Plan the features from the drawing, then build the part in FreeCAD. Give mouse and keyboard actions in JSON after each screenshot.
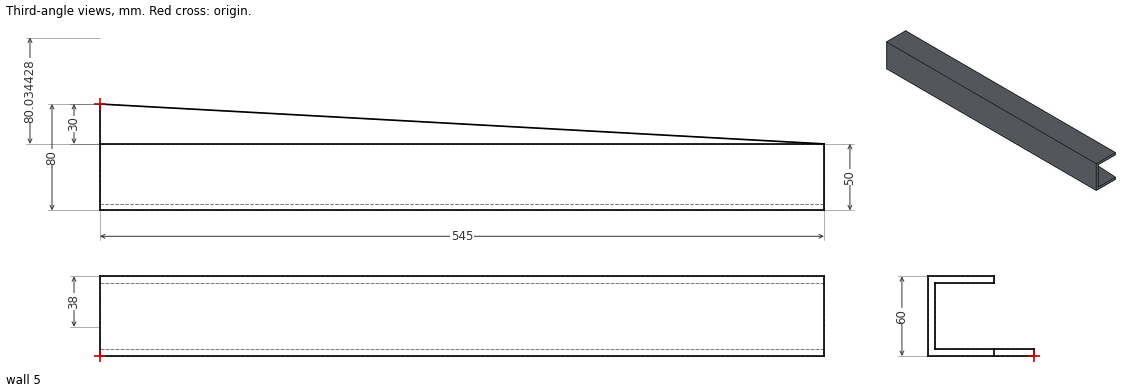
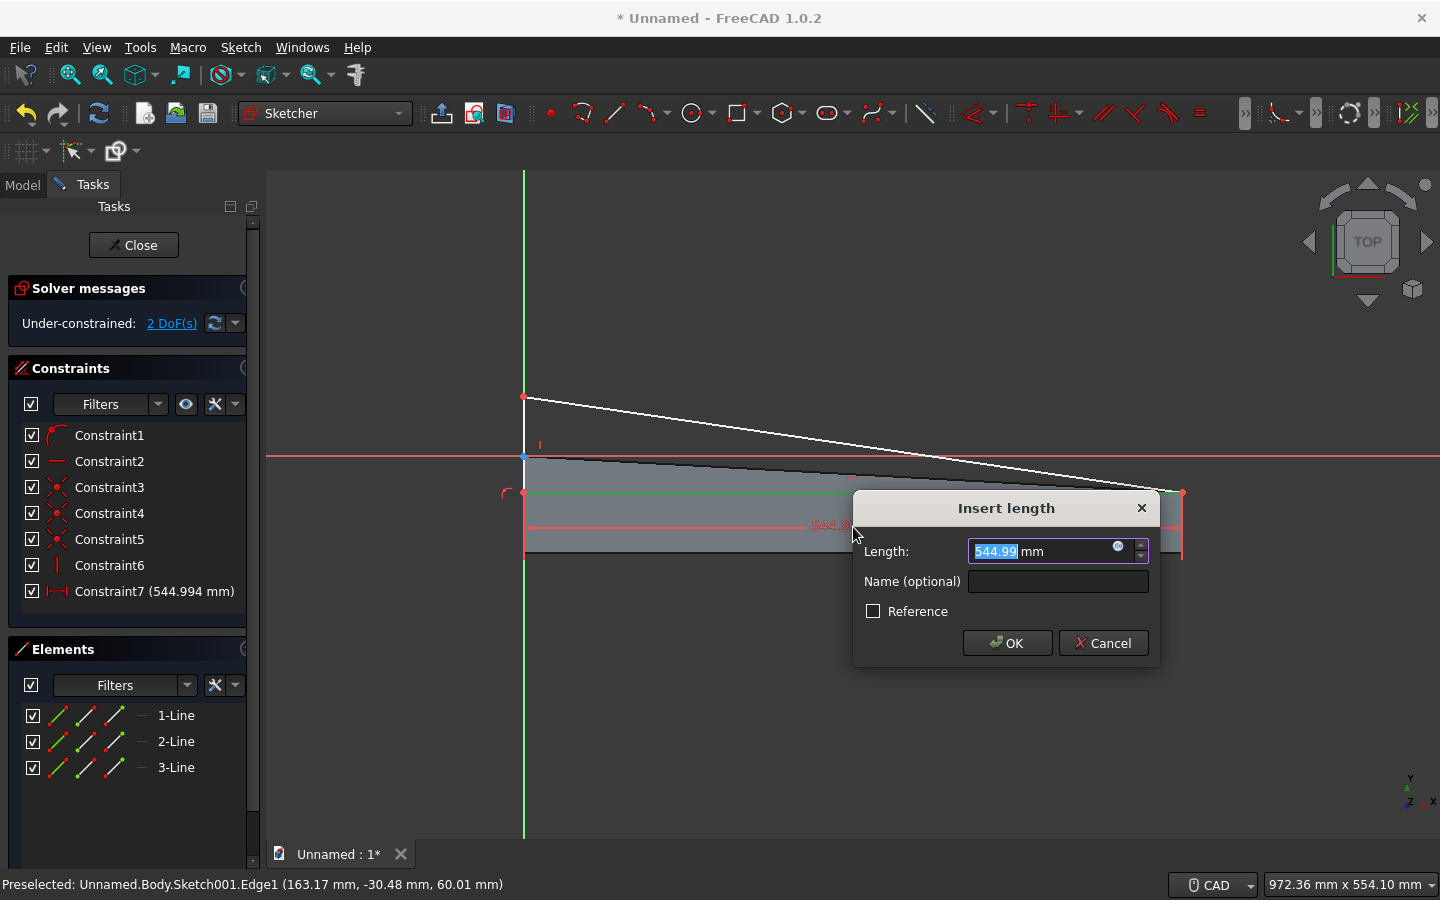
{"action": "type", "text": "545"}
{"action": "key", "text": "Return"}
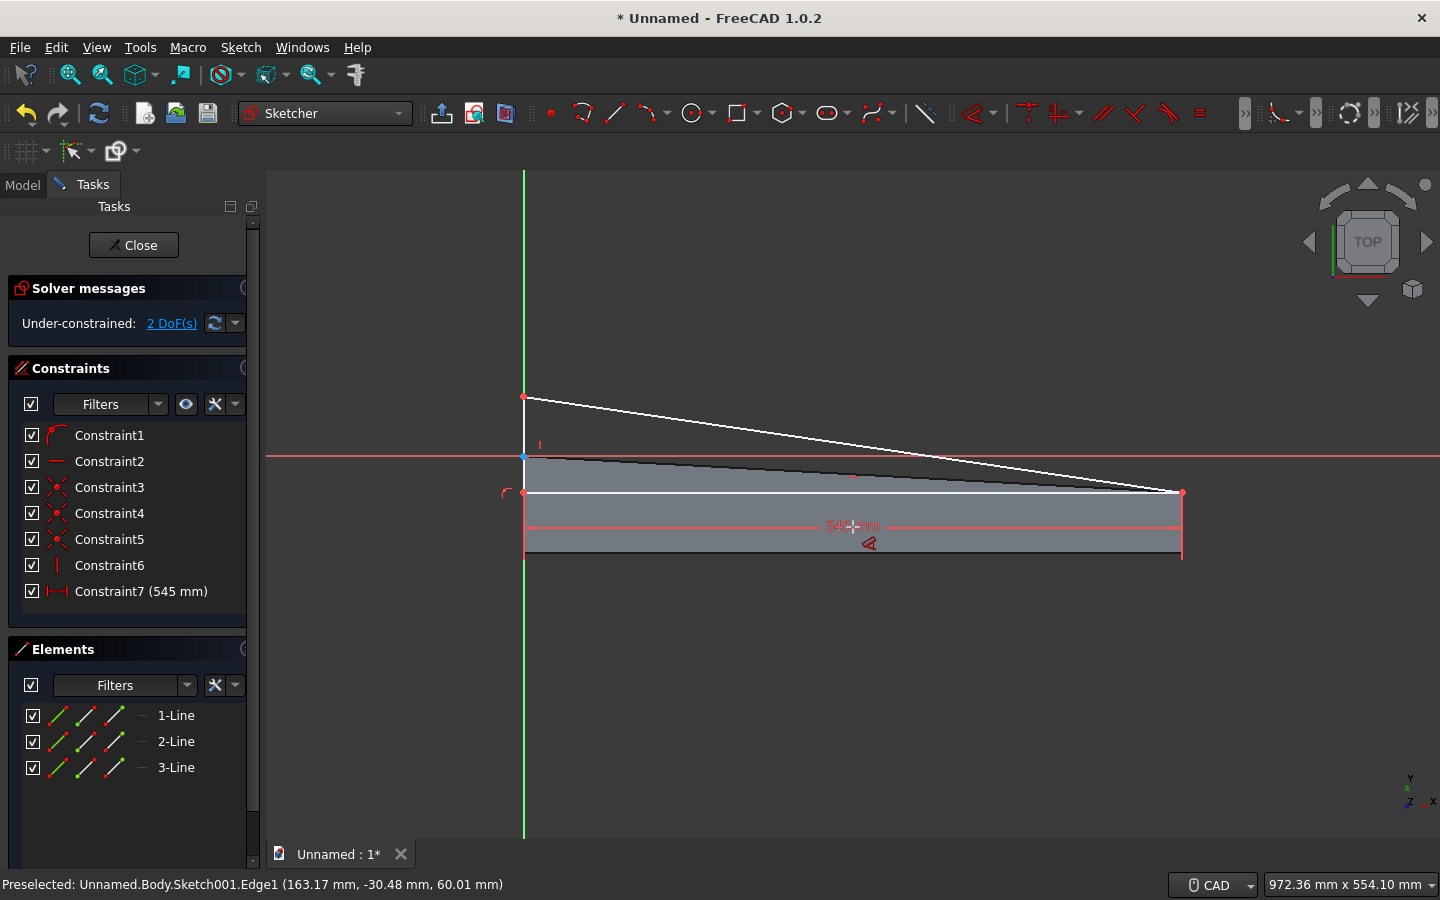
{"action": "left_click", "coordinate": [524, 493]}
{"action": "left_click", "coordinate": [490, 475]}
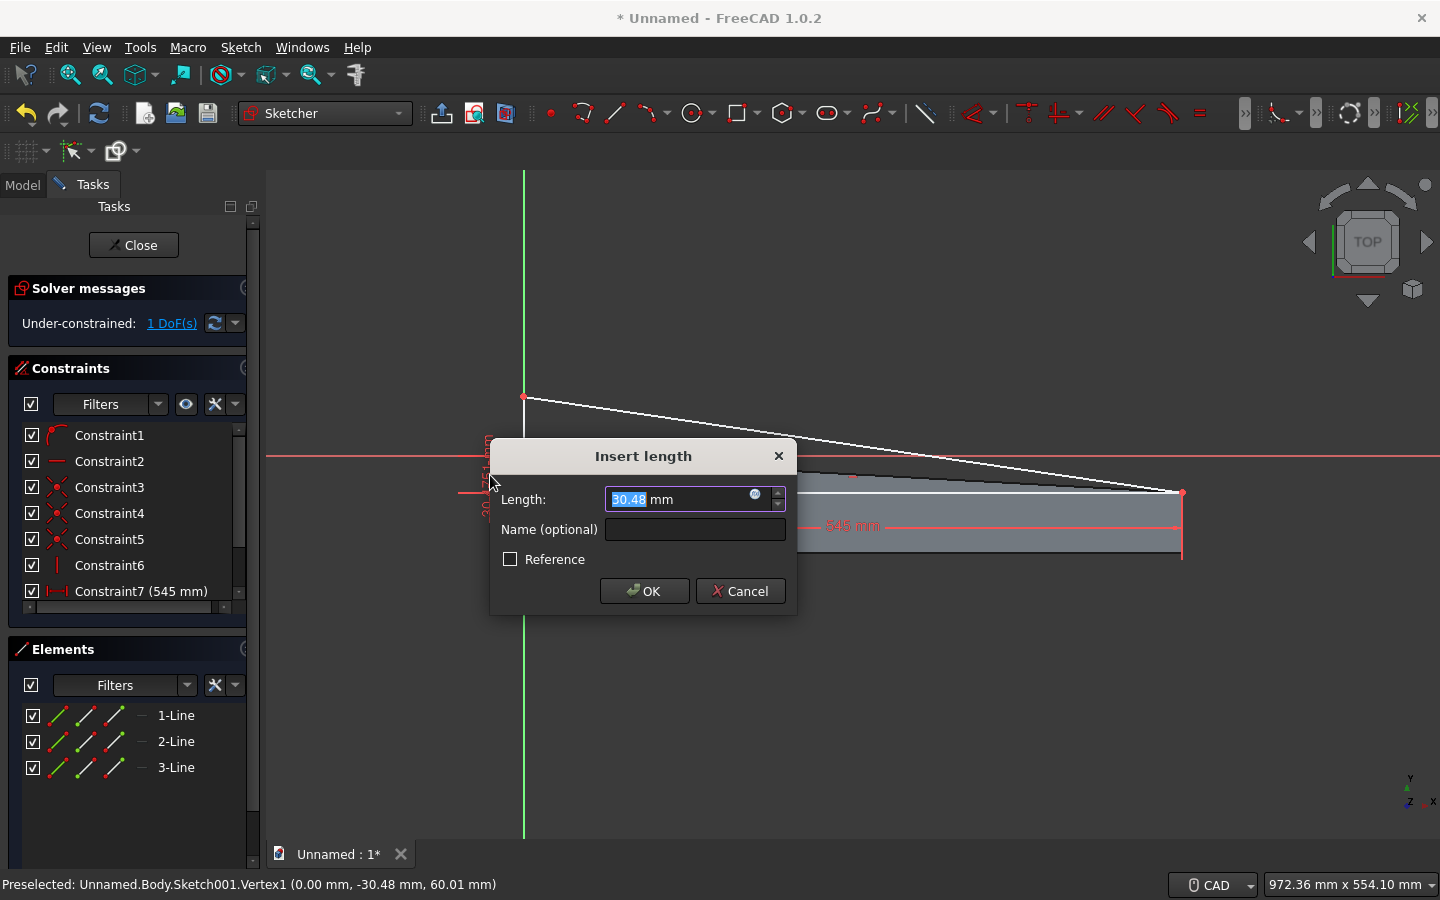
{"action": "type", "text": "30"}
{"action": "key", "text": "Return"}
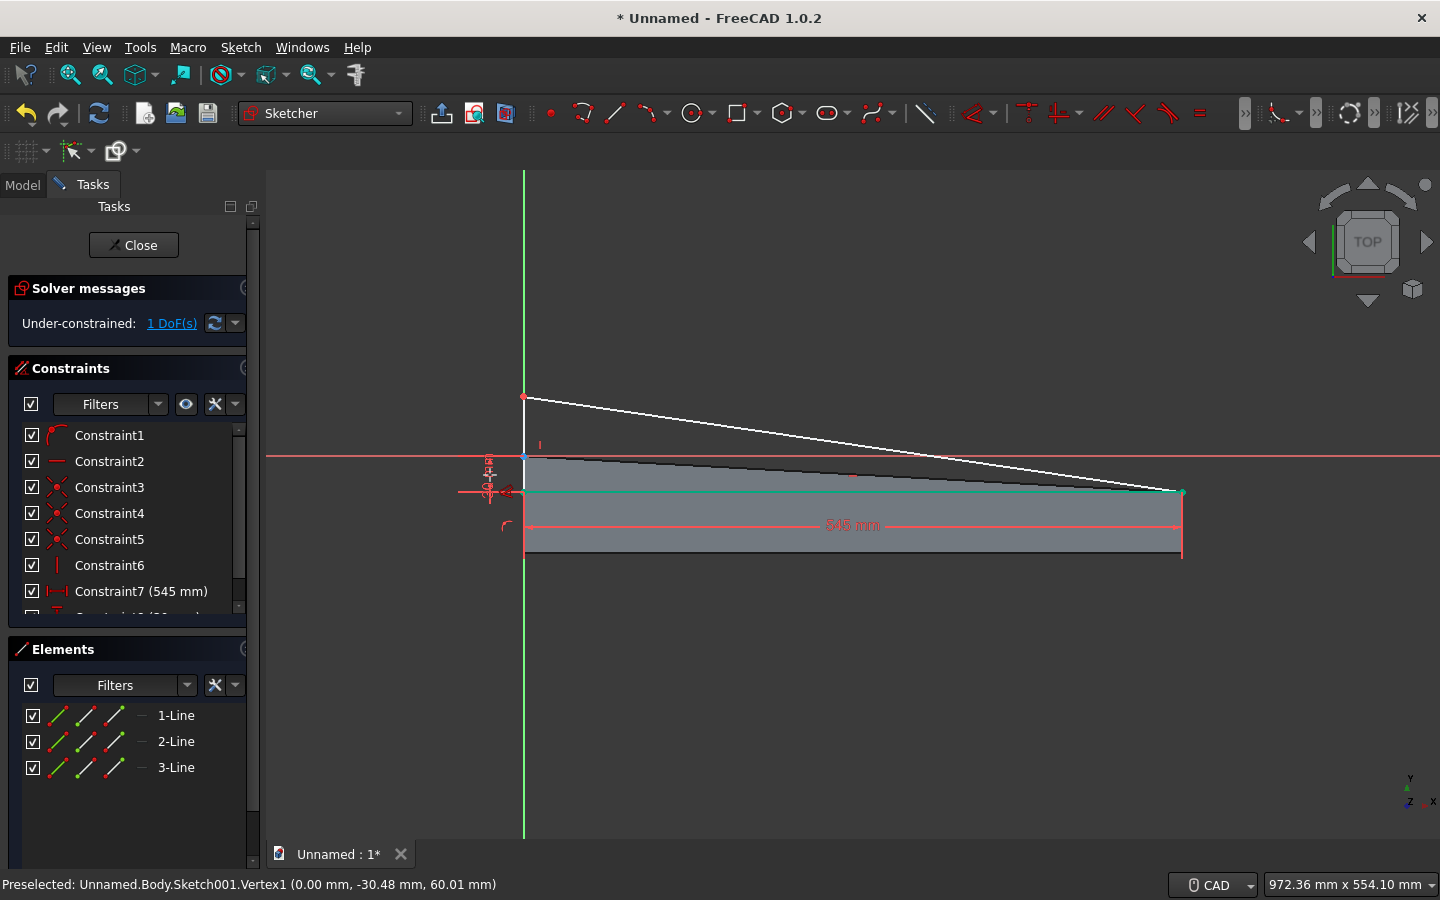
{"action": "left_click", "coordinate": [524, 426]}
{"action": "left_click", "coordinate": [490, 423]}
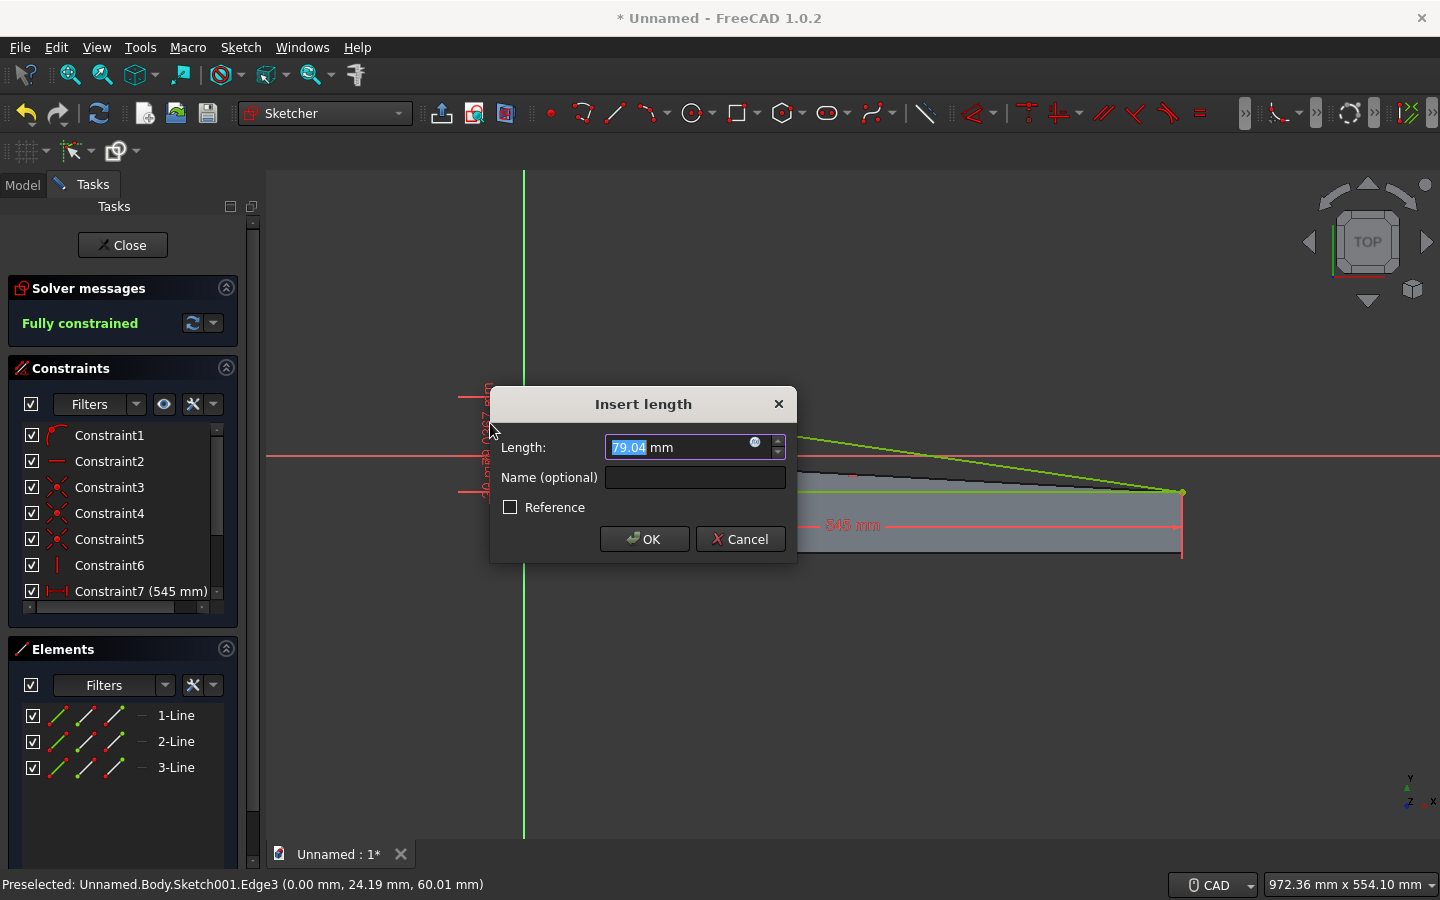
{"action": "type", "text": "80.034428"}
{"action": "key", "text": "Return"}
{"action": "key", "text": "Escape"}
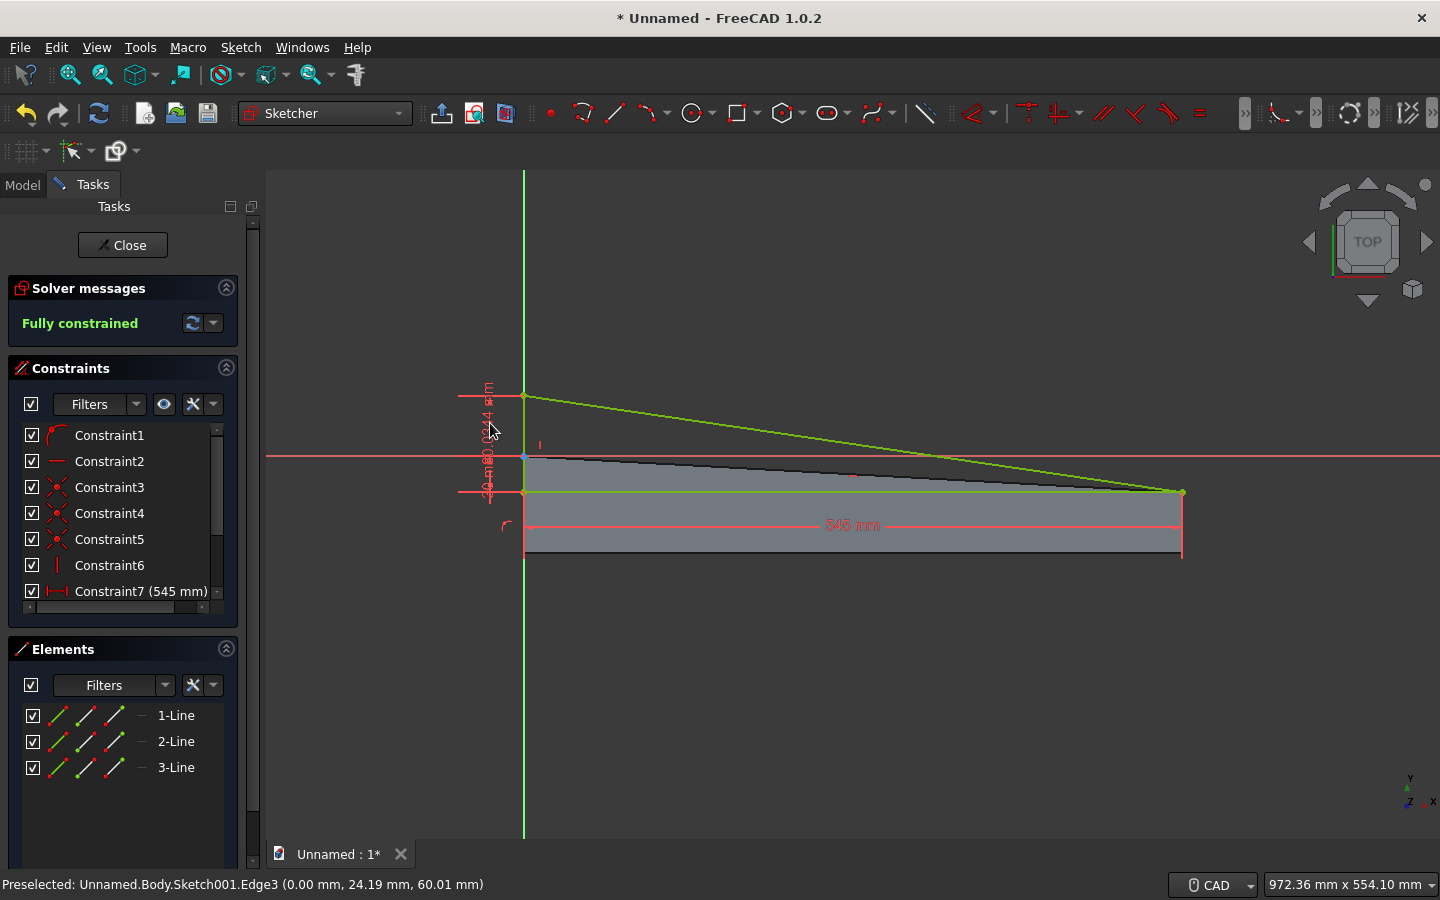
{"action": "left_click", "coordinate": [123, 245]}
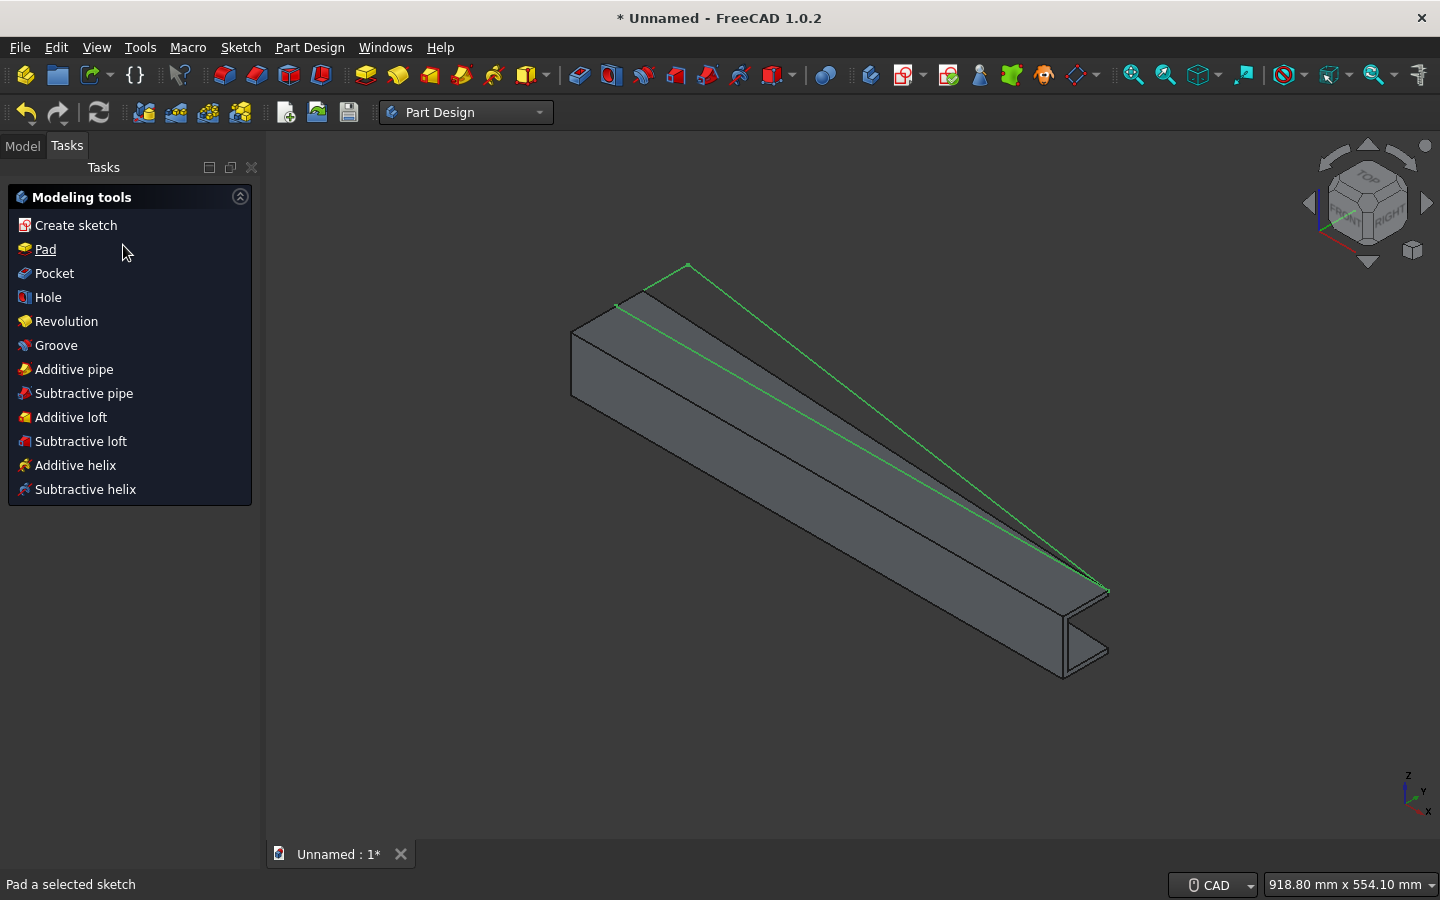
{"action": "left_click", "coordinate": [580, 76]}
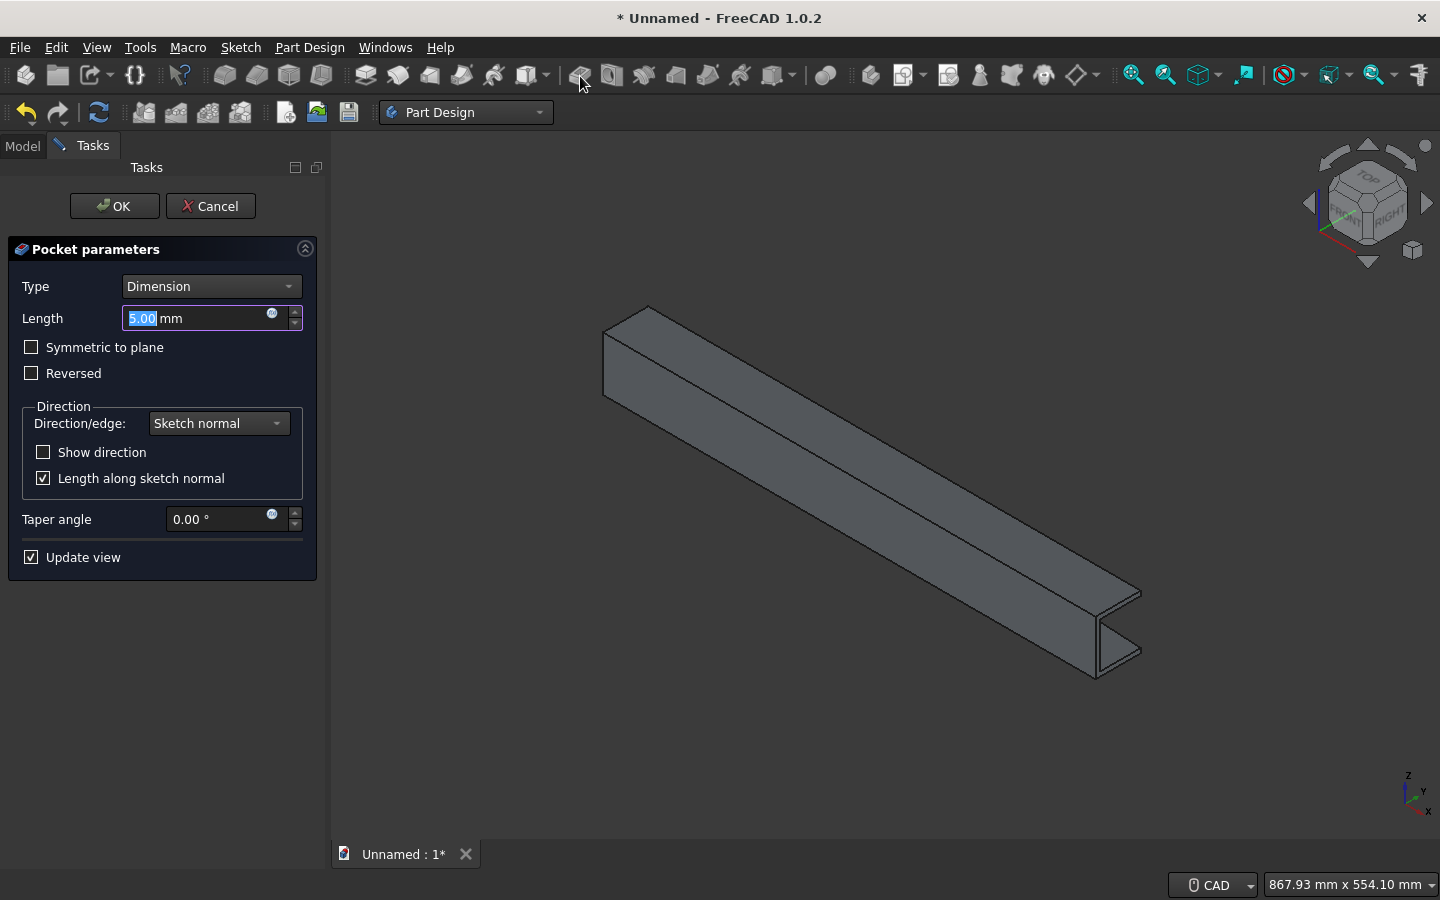
{"action": "type", "text": "38"}
{"action": "key", "text": "Tab"}